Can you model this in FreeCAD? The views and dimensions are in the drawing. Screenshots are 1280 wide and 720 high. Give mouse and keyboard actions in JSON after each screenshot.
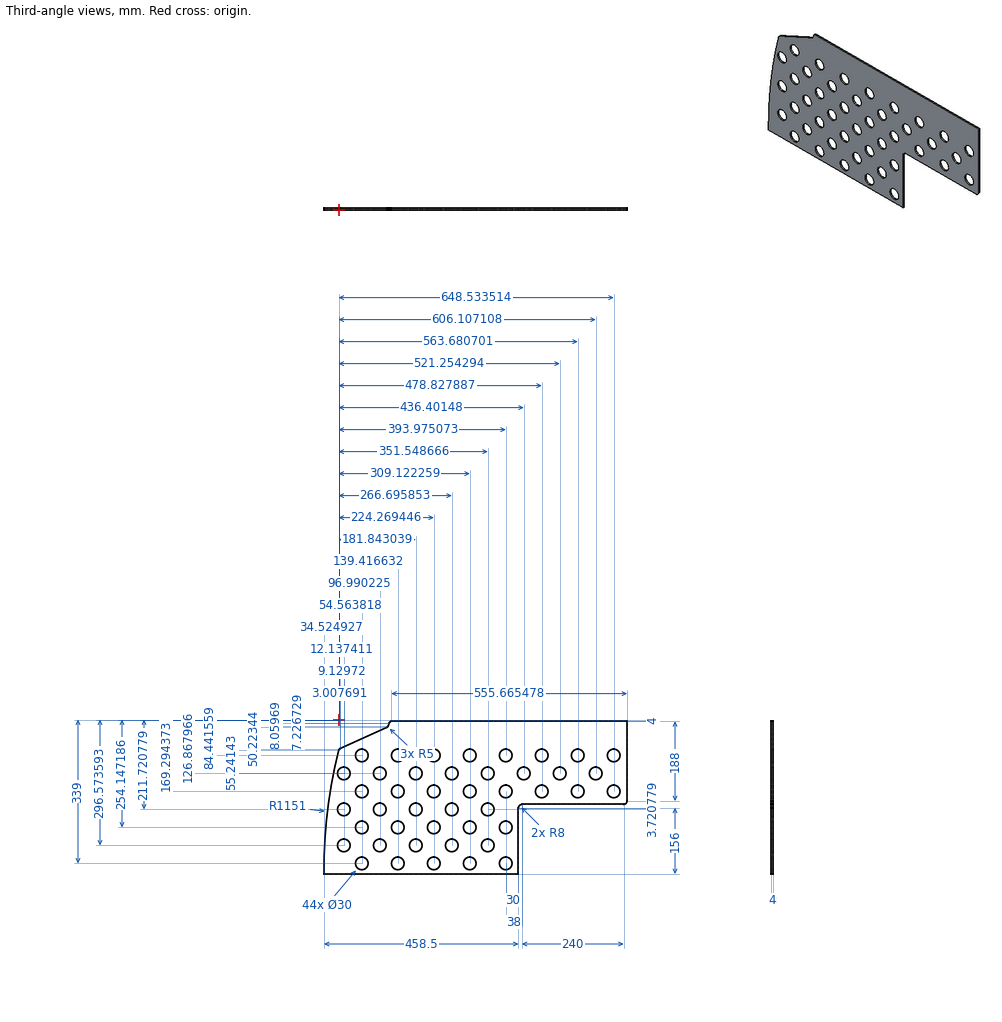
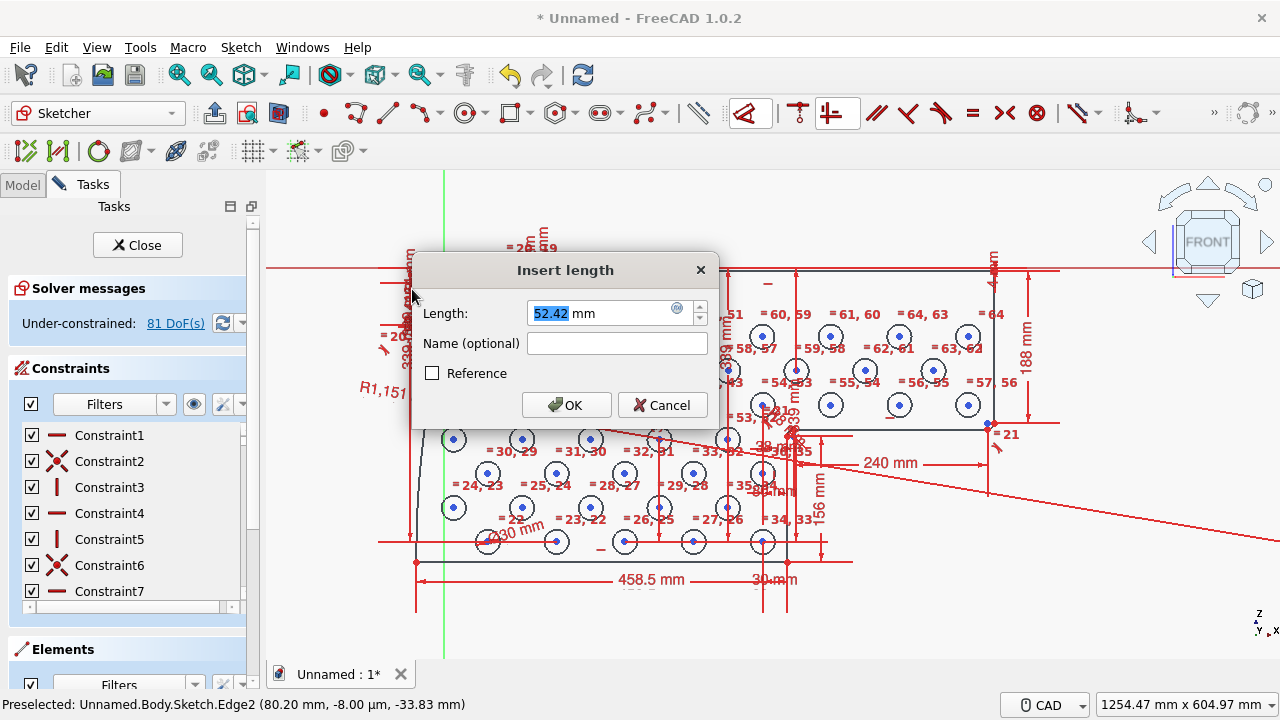
{"action": "type", "text": "50.22344"}
{"action": "key", "text": "Return"}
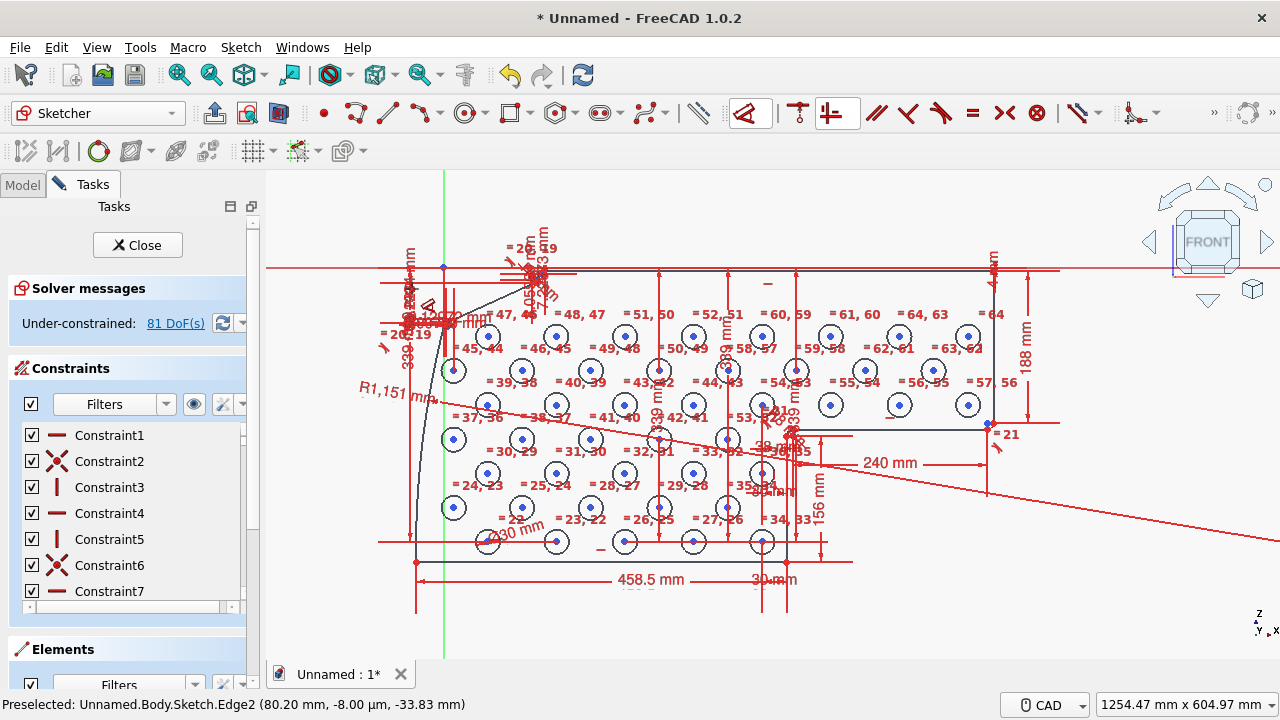
{"action": "left_click", "coordinate": [488, 542]}
{"action": "left_click", "coordinate": [466, 234]}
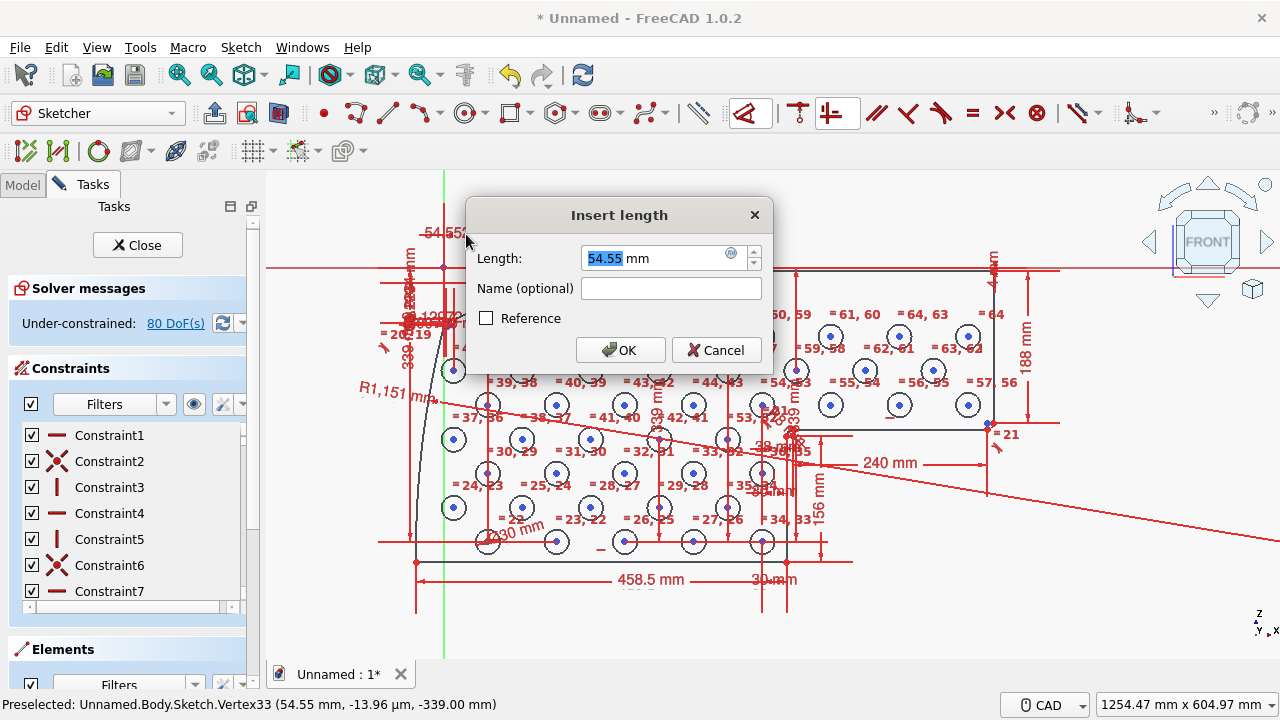
{"action": "type", "text": "54.563818"}
{"action": "key", "text": "Return"}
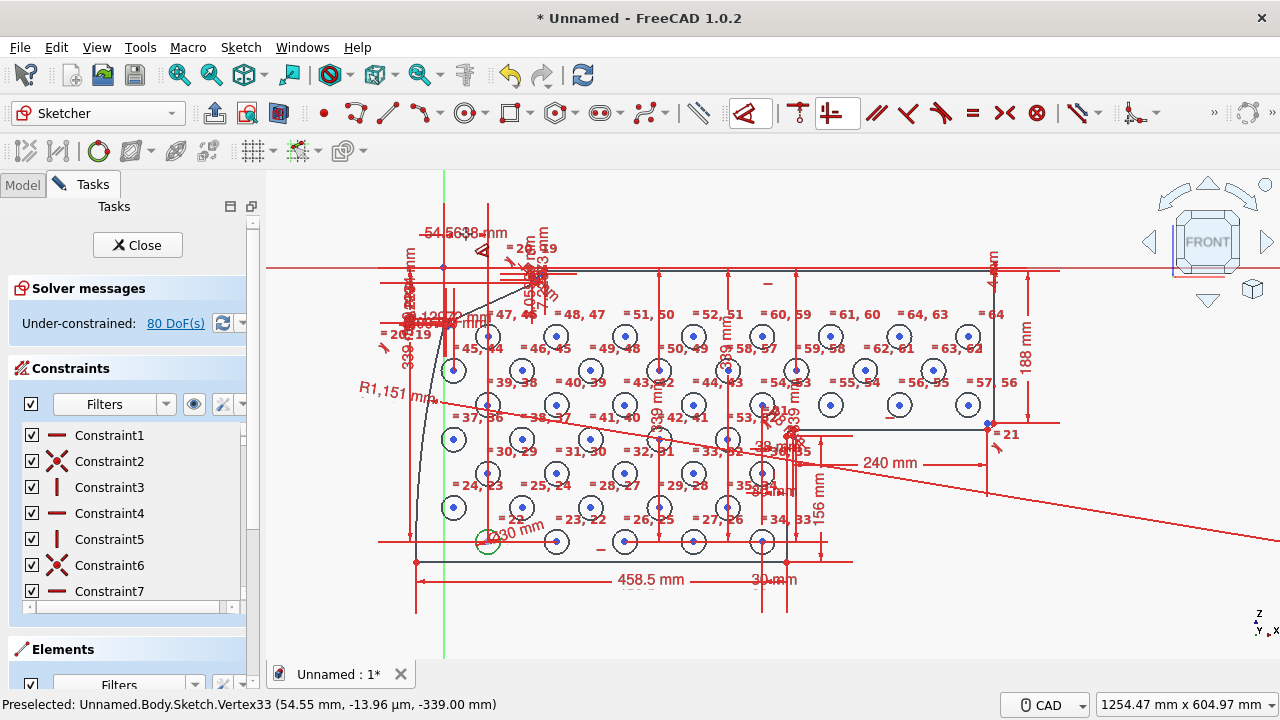
{"action": "scroll", "coordinate": [454, 508], "scroll_direction": "up", "scroll_amount": 7}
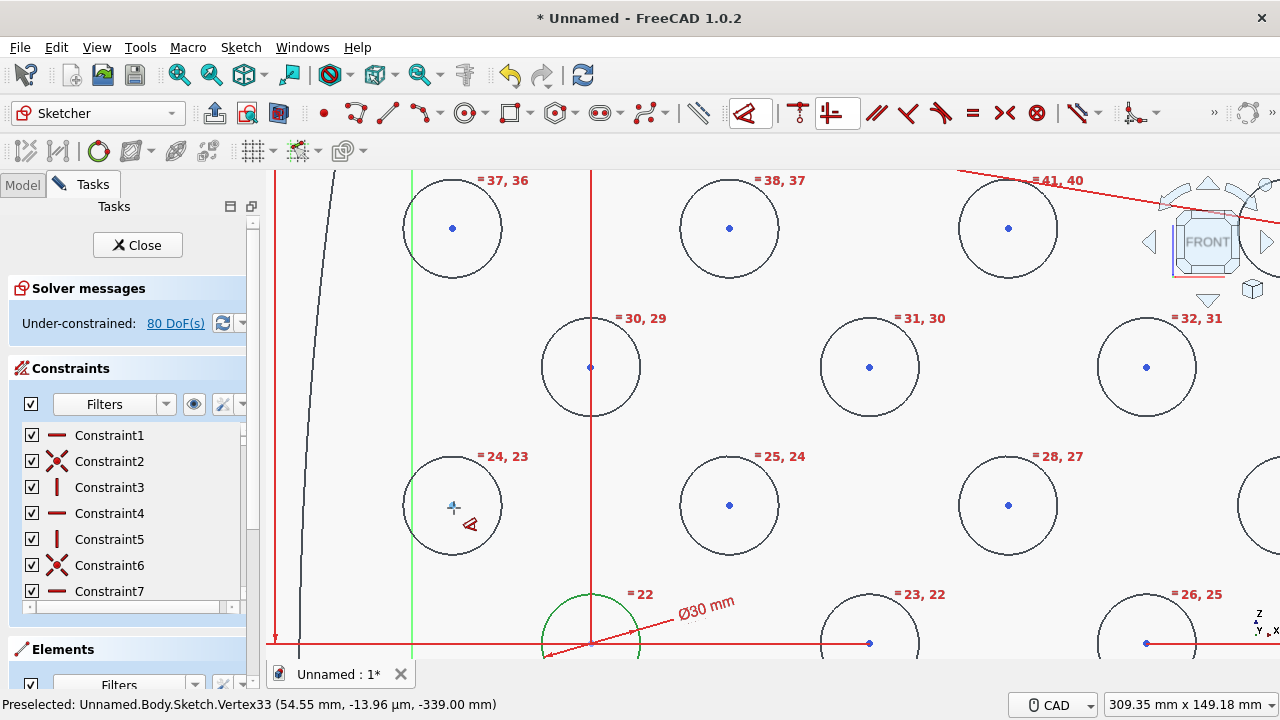
{"action": "left_click", "coordinate": [453, 506]}
{"action": "left_click", "coordinate": [442, 540]}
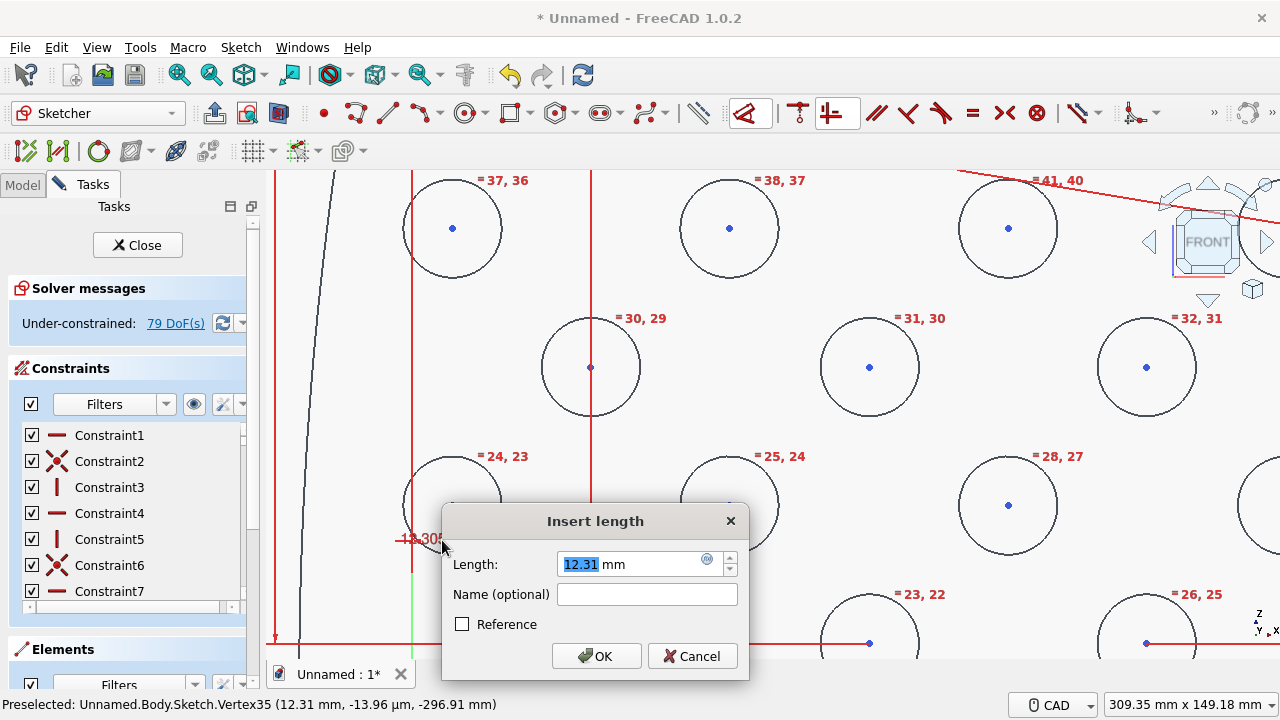
{"action": "type", "text": "12.137411"}
{"action": "key", "text": "Return"}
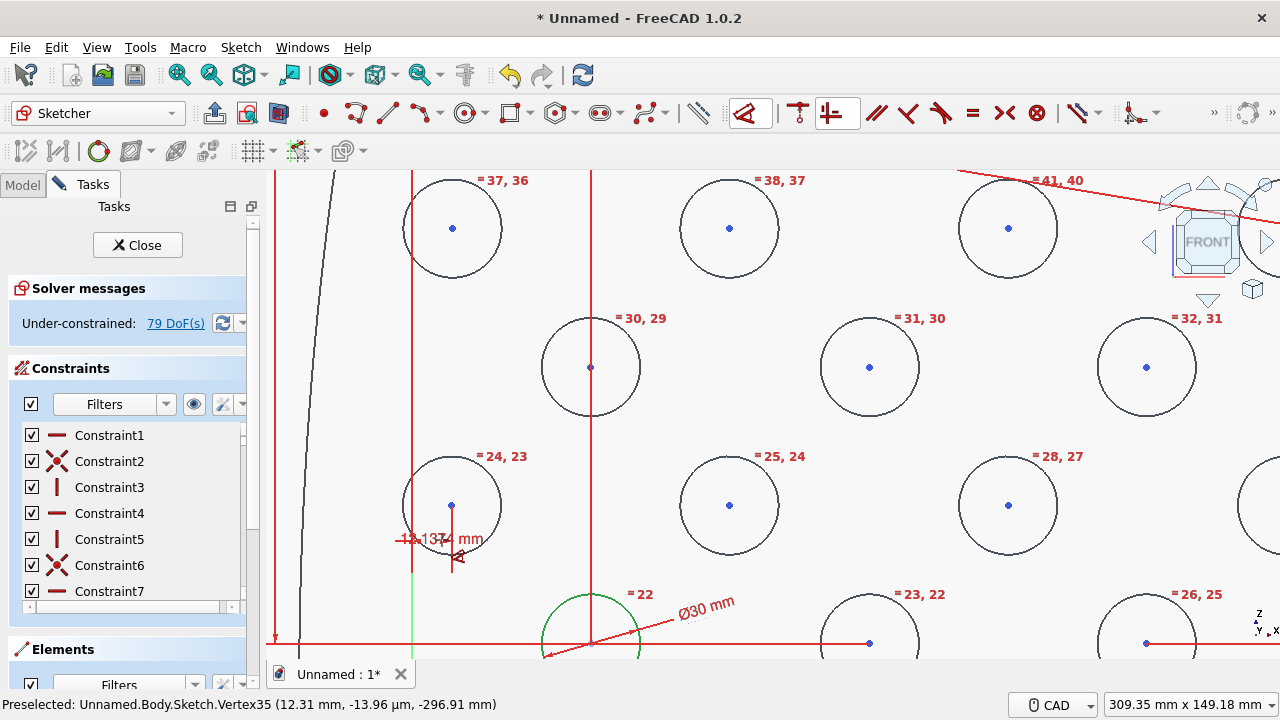
{"action": "scroll", "coordinate": [454, 508], "scroll_direction": "down", "scroll_amount": 7}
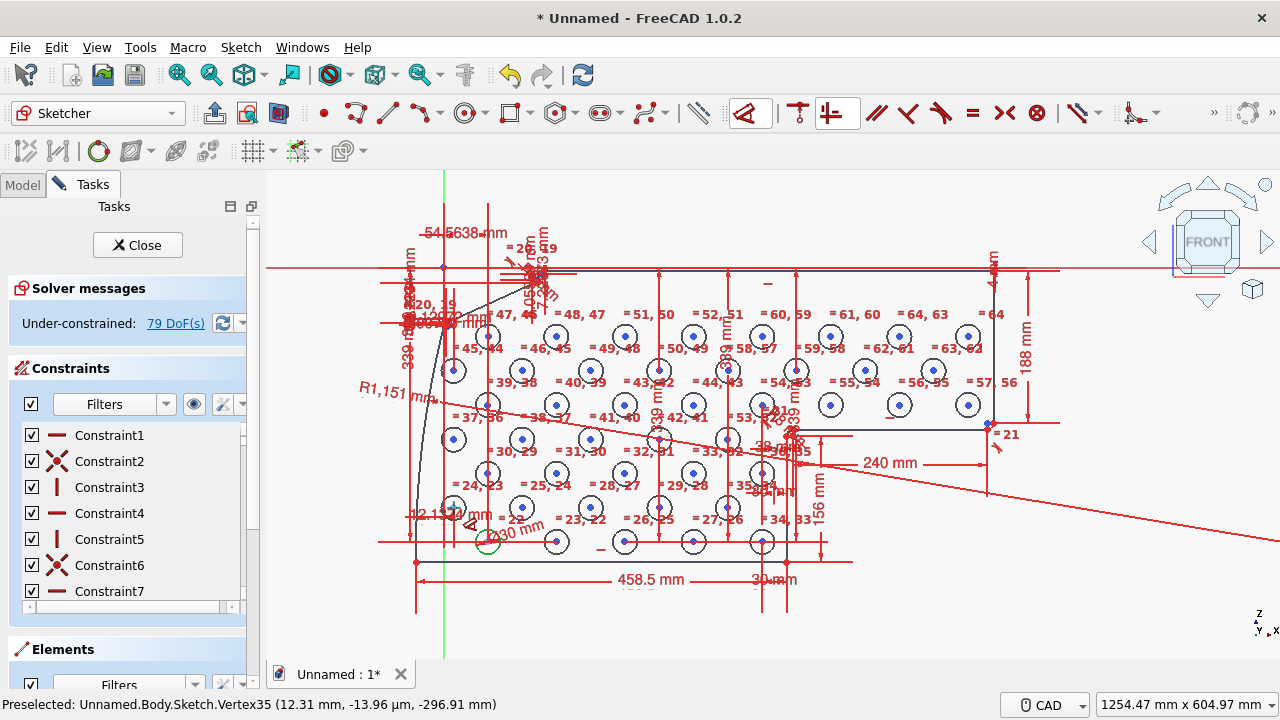
{"action": "left_click", "coordinate": [522, 508]}
{"action": "left_click", "coordinate": [483, 210]}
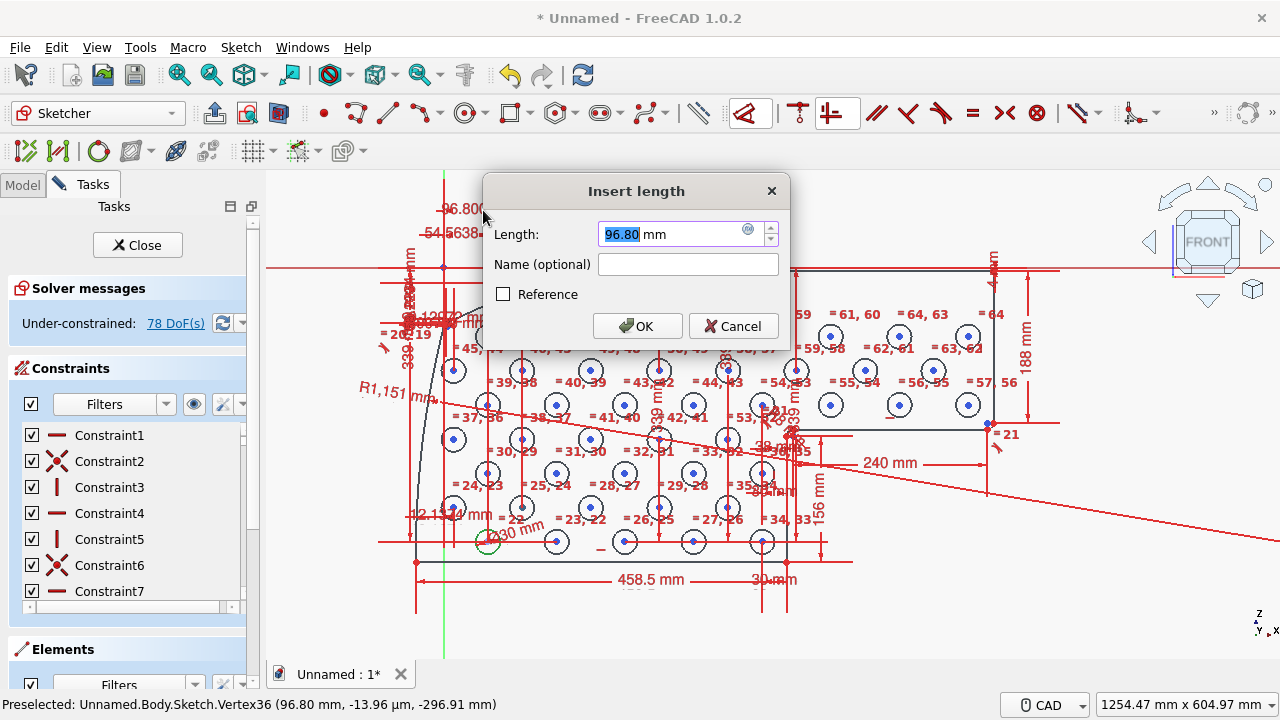
{"action": "type", "text": "96.990225"}
{"action": "key", "text": "Return"}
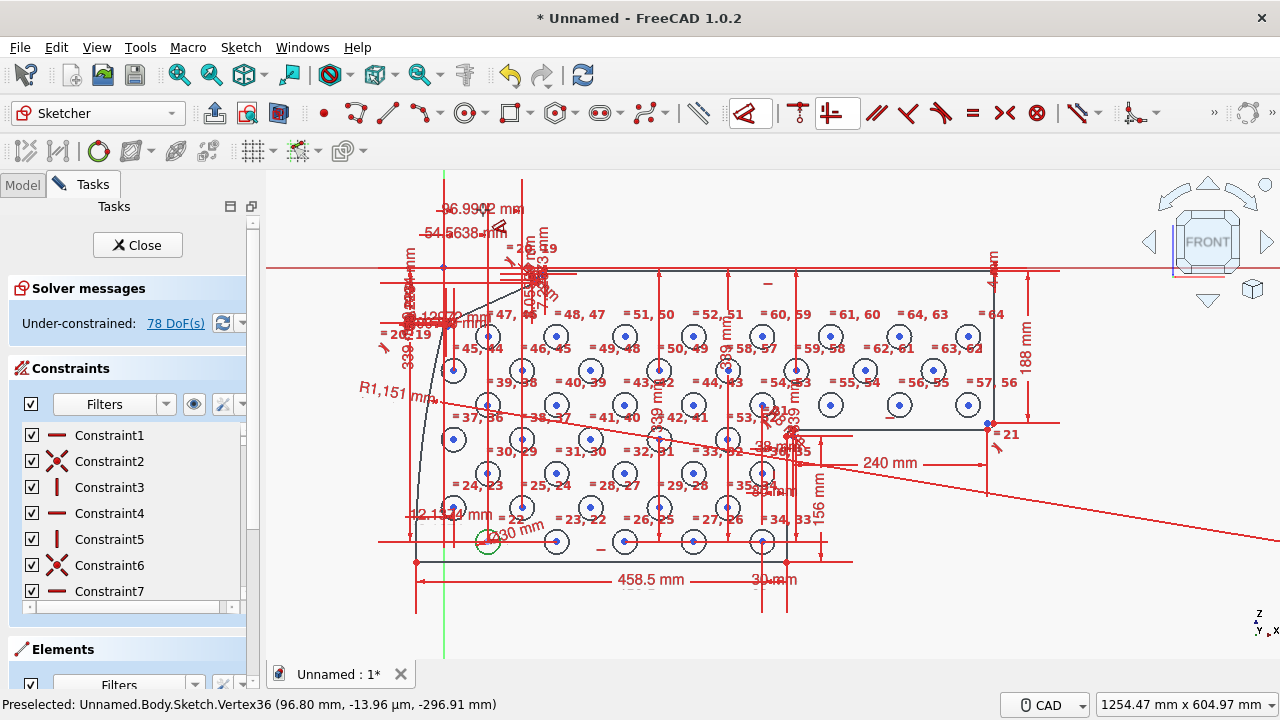
{"action": "left_click", "coordinate": [488, 474]}
{"action": "left_click", "coordinate": [466, 580]}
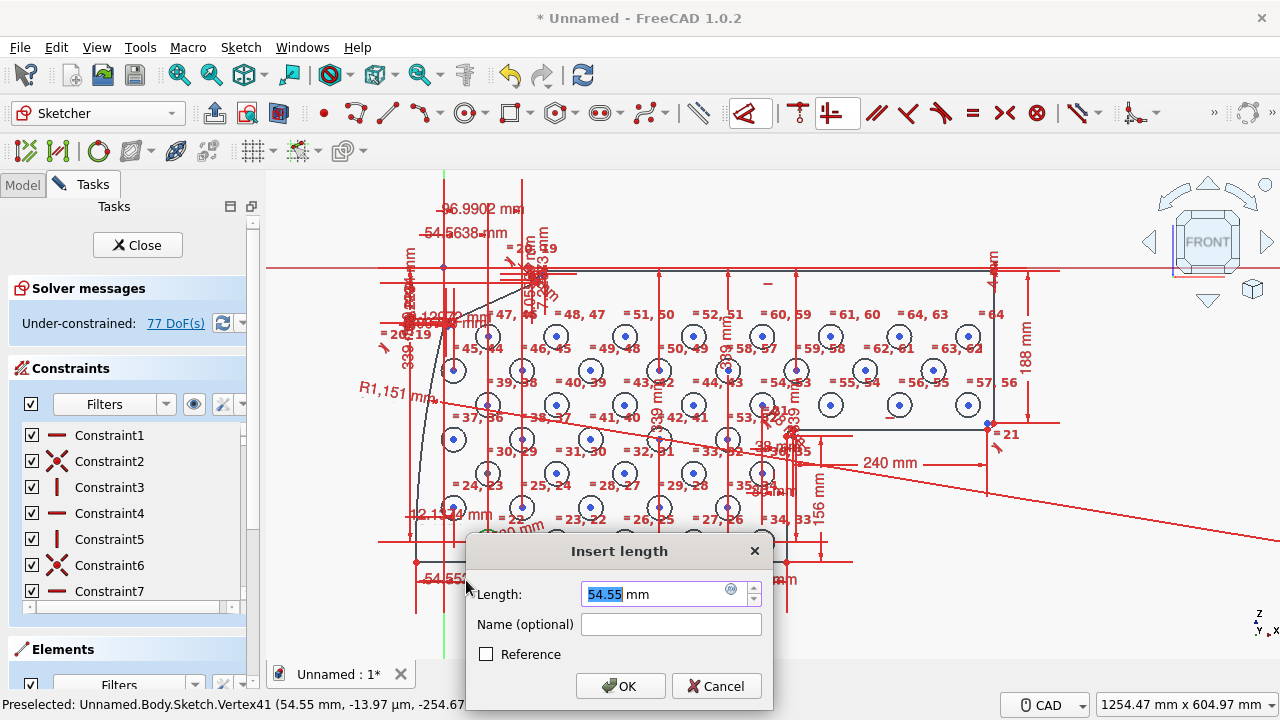
{"action": "type", "text": "54.563818"}
{"action": "key", "text": "Return"}